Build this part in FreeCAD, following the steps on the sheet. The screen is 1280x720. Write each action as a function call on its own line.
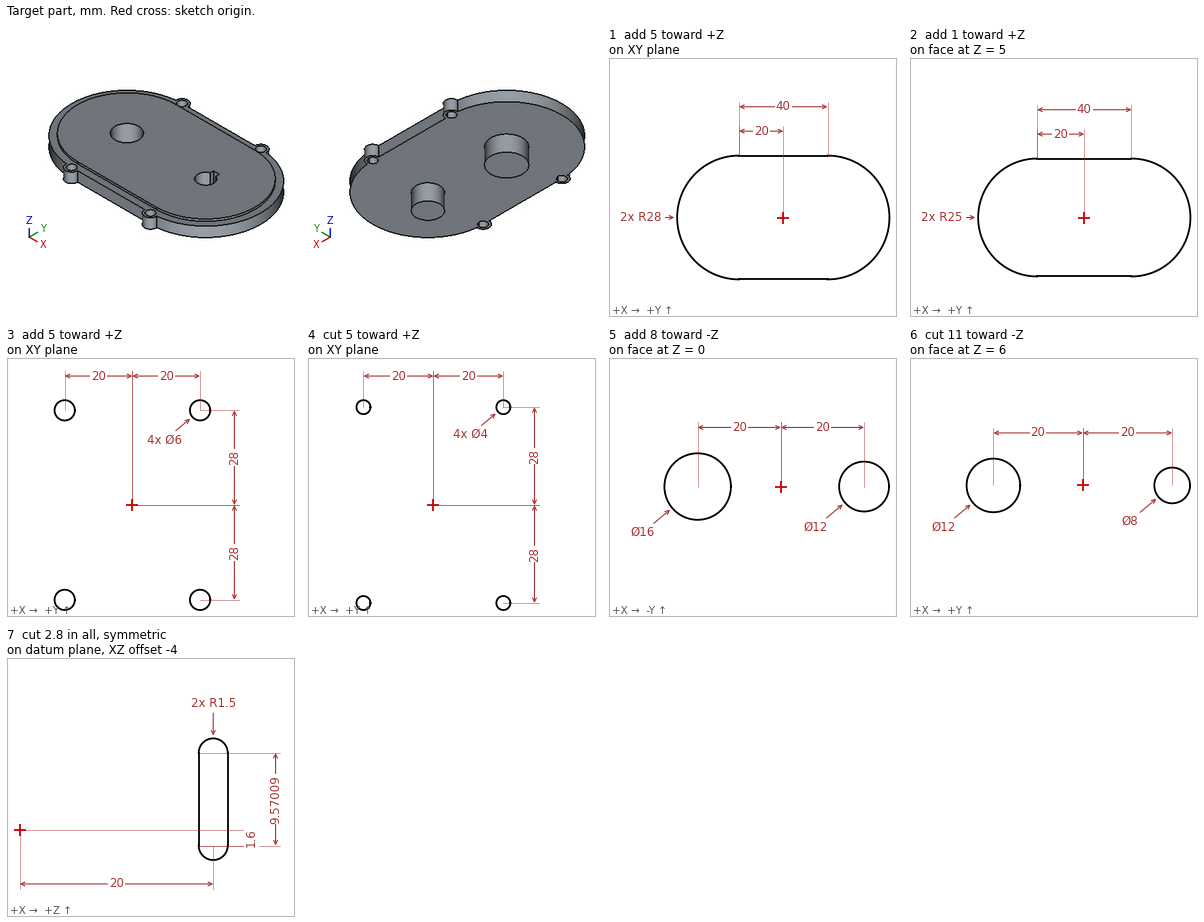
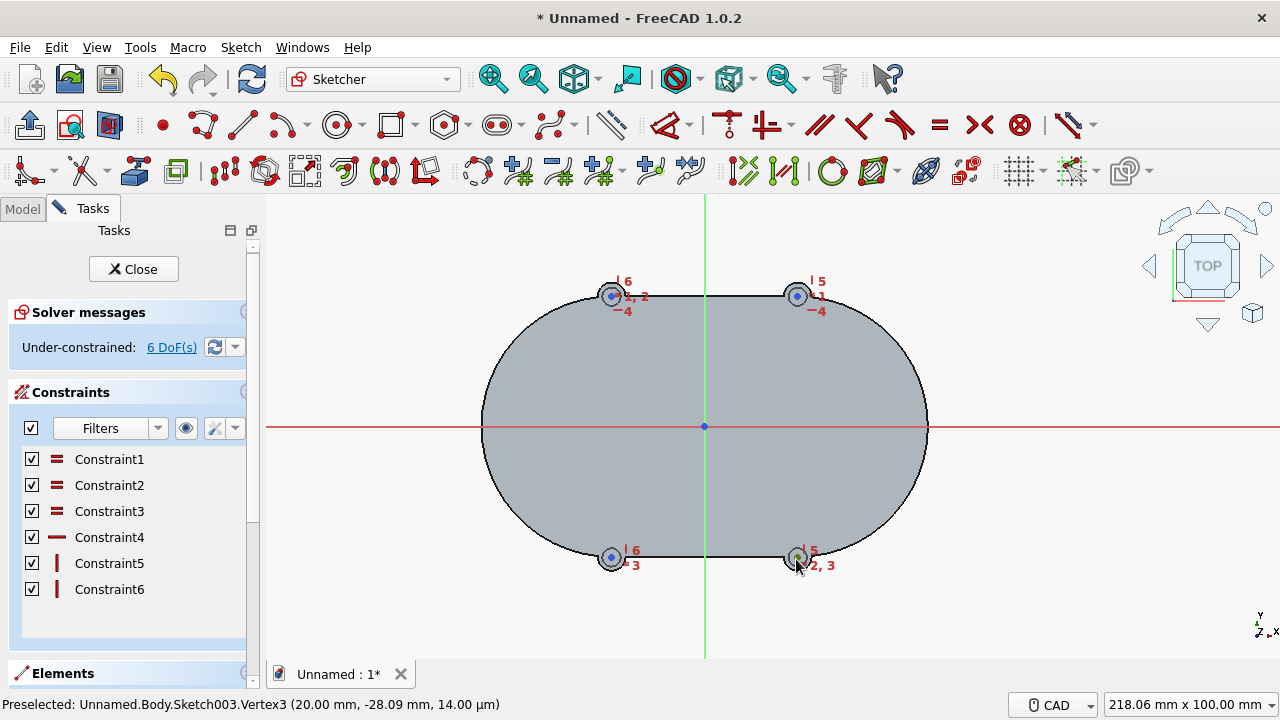
click(612, 557)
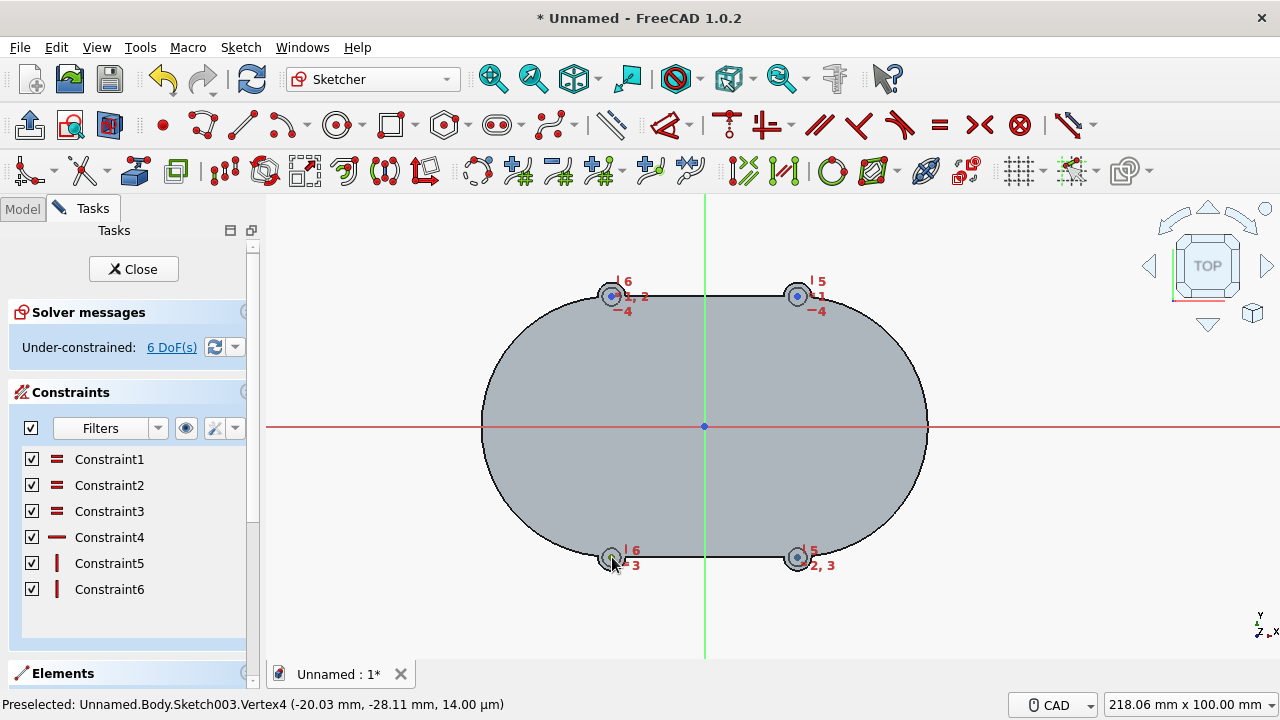
key(h)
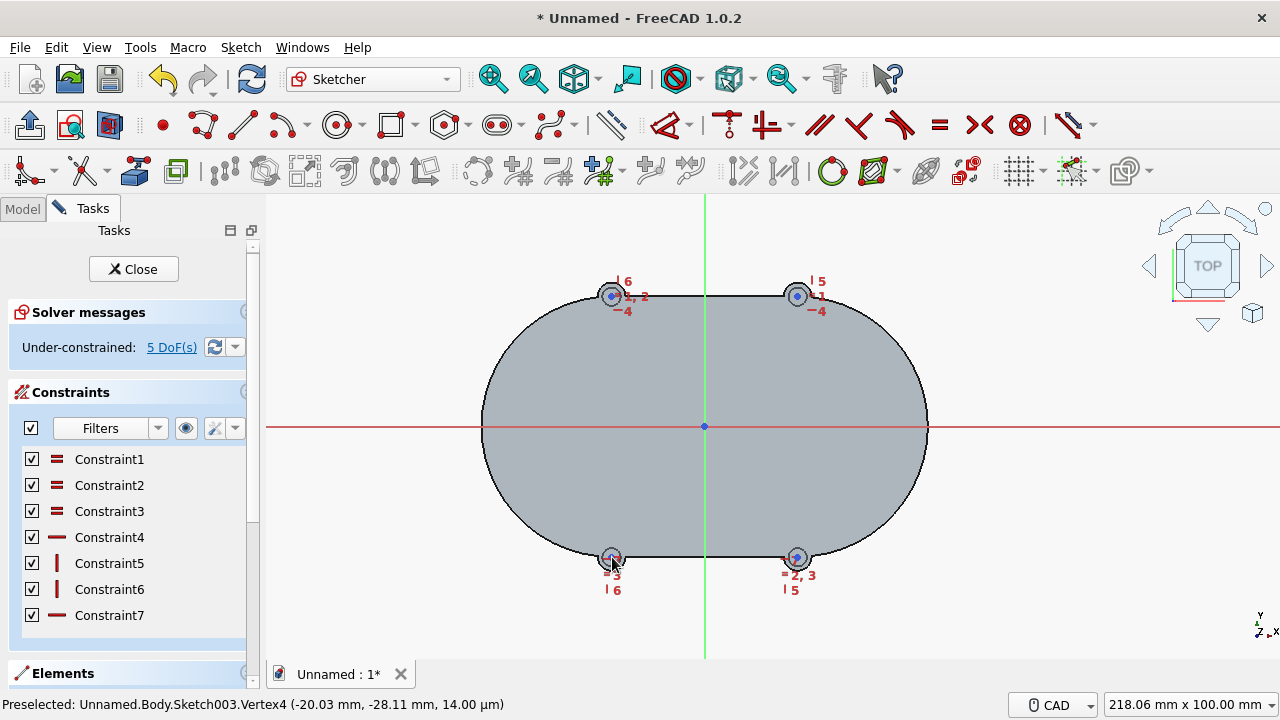
key(d)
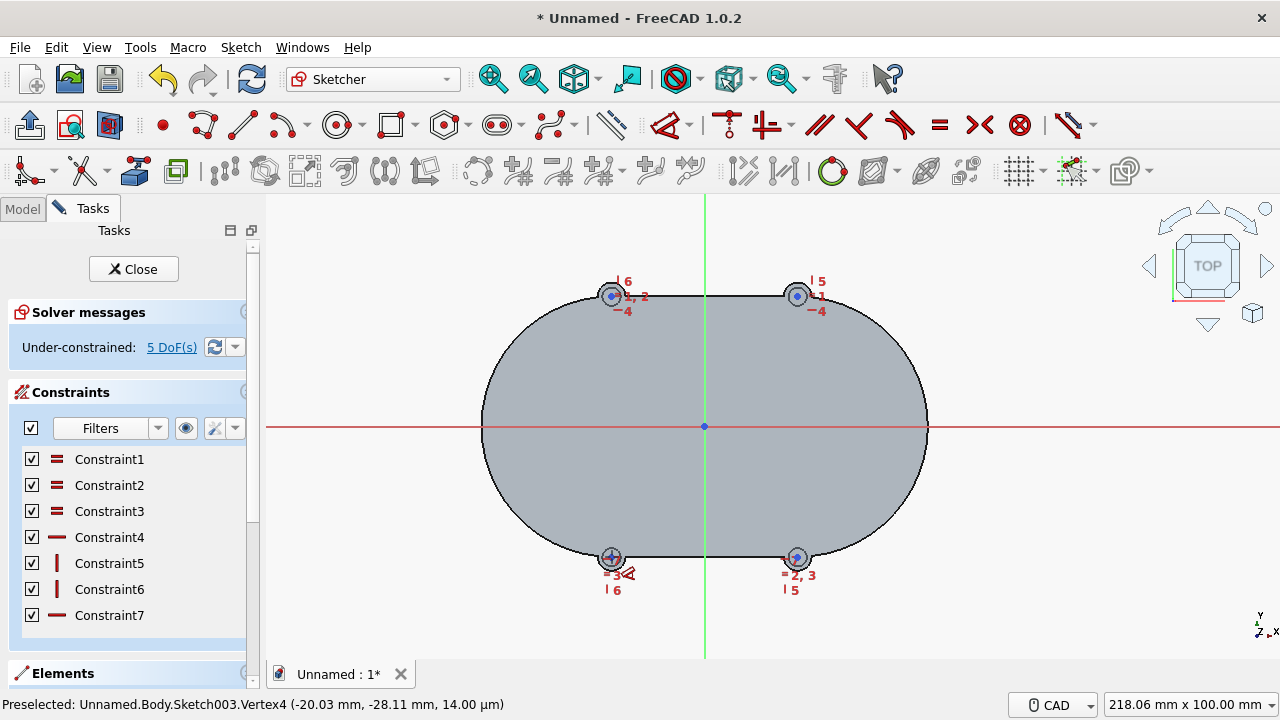
scroll(804, 290, up, 4)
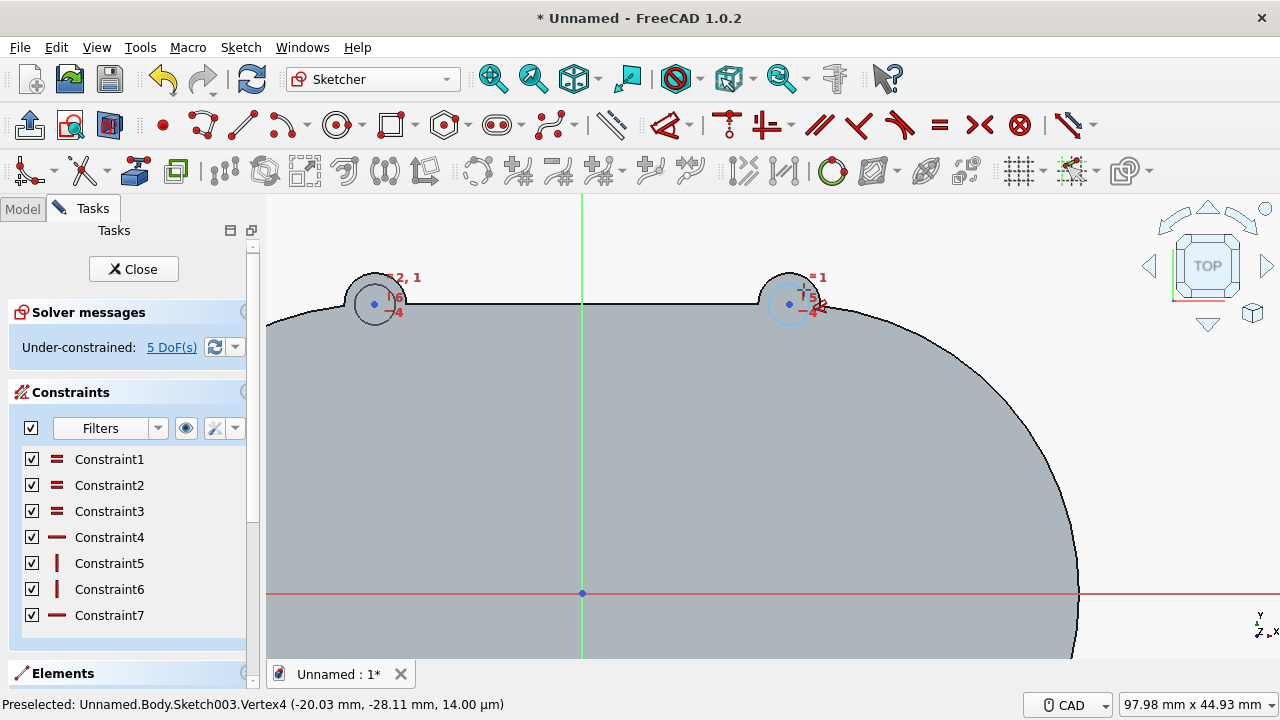
click(804, 290)
click(827, 267)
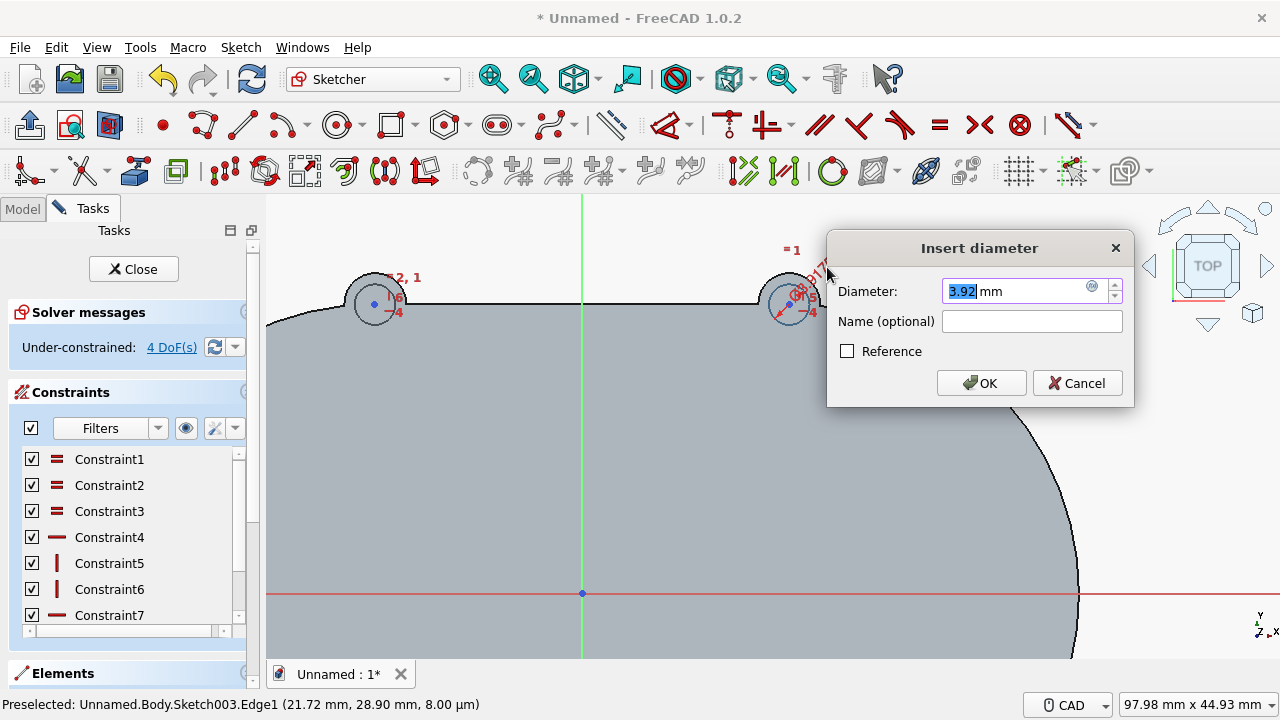
text(4)
key(Return)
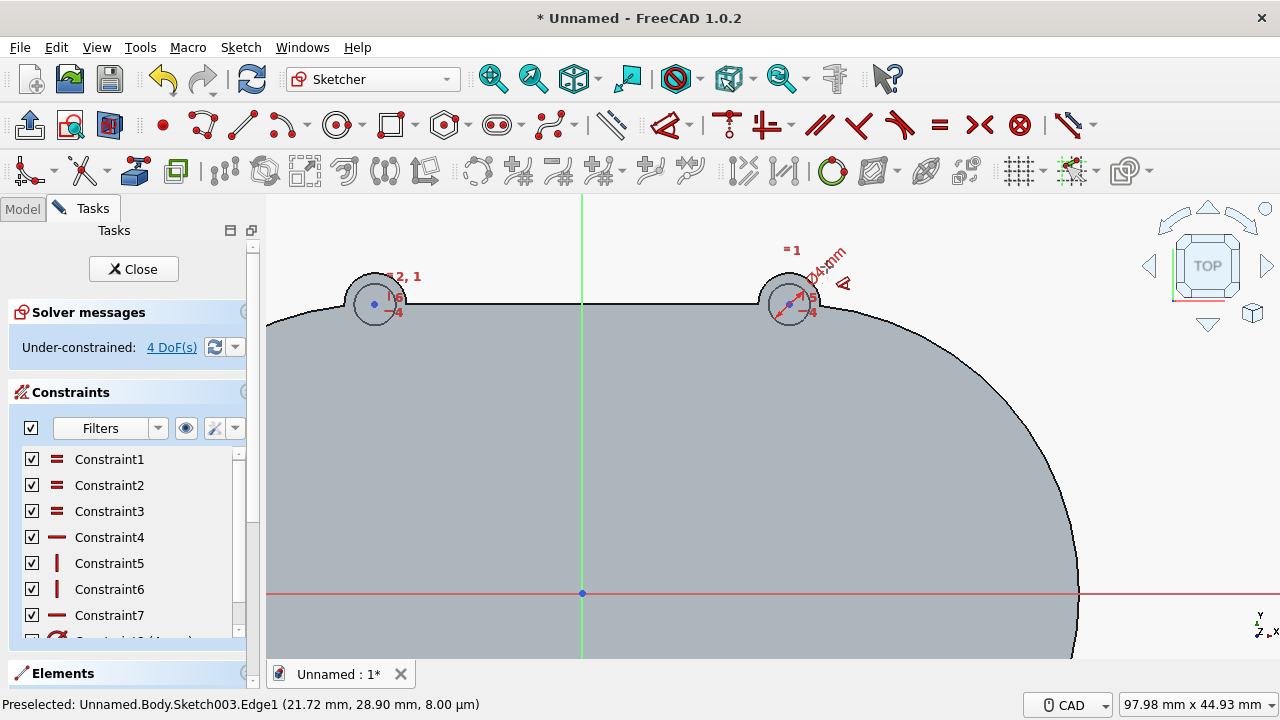
click(789, 305)
click(686, 271)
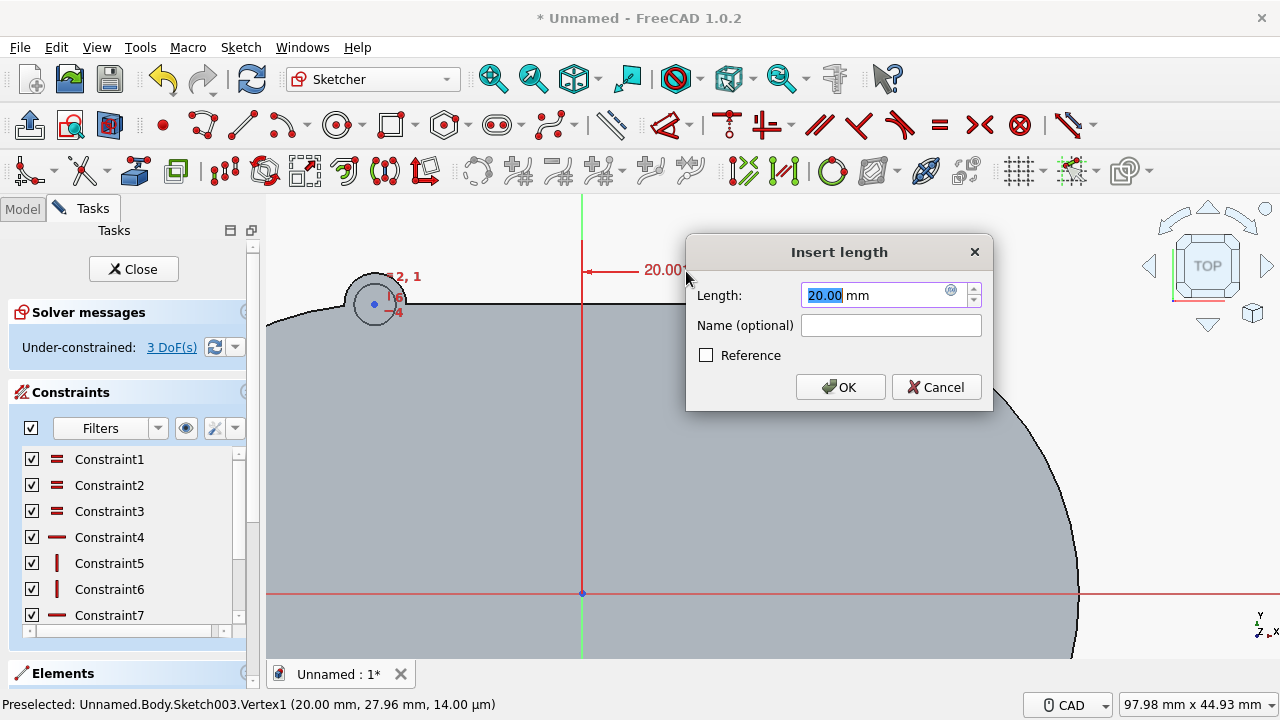
text(20)
key(Return)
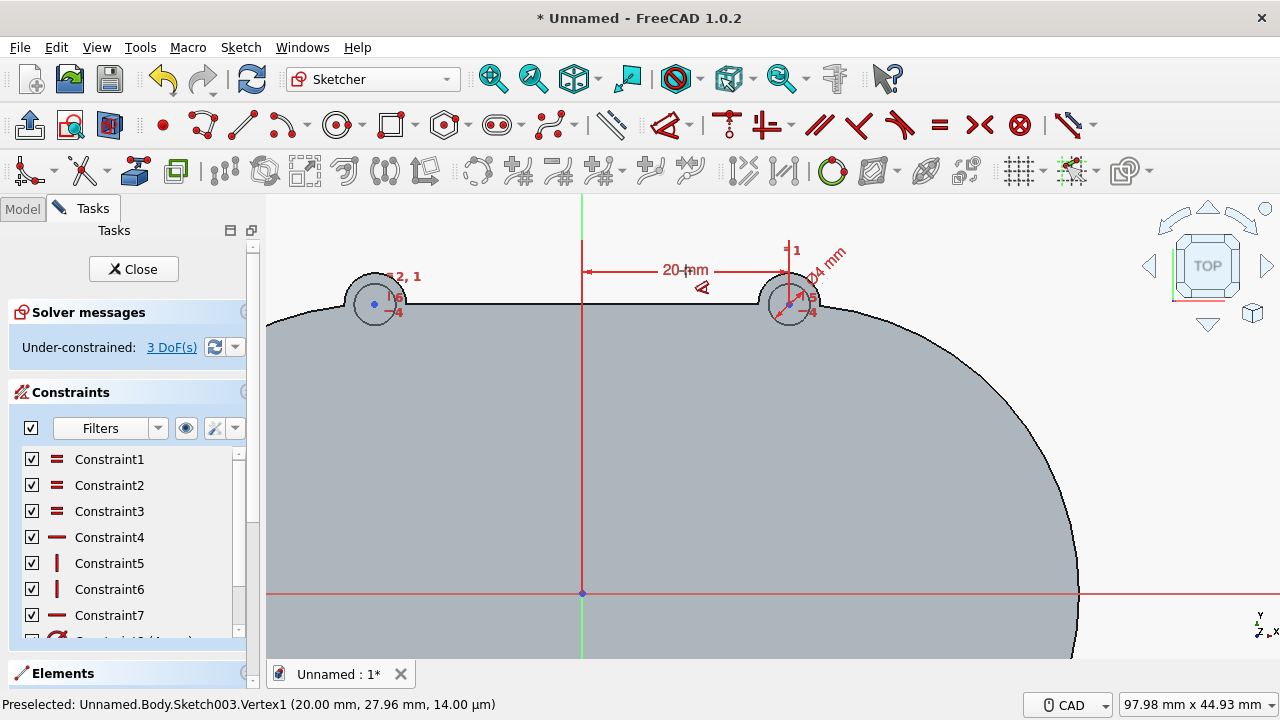
click(789, 305)
click(823, 449)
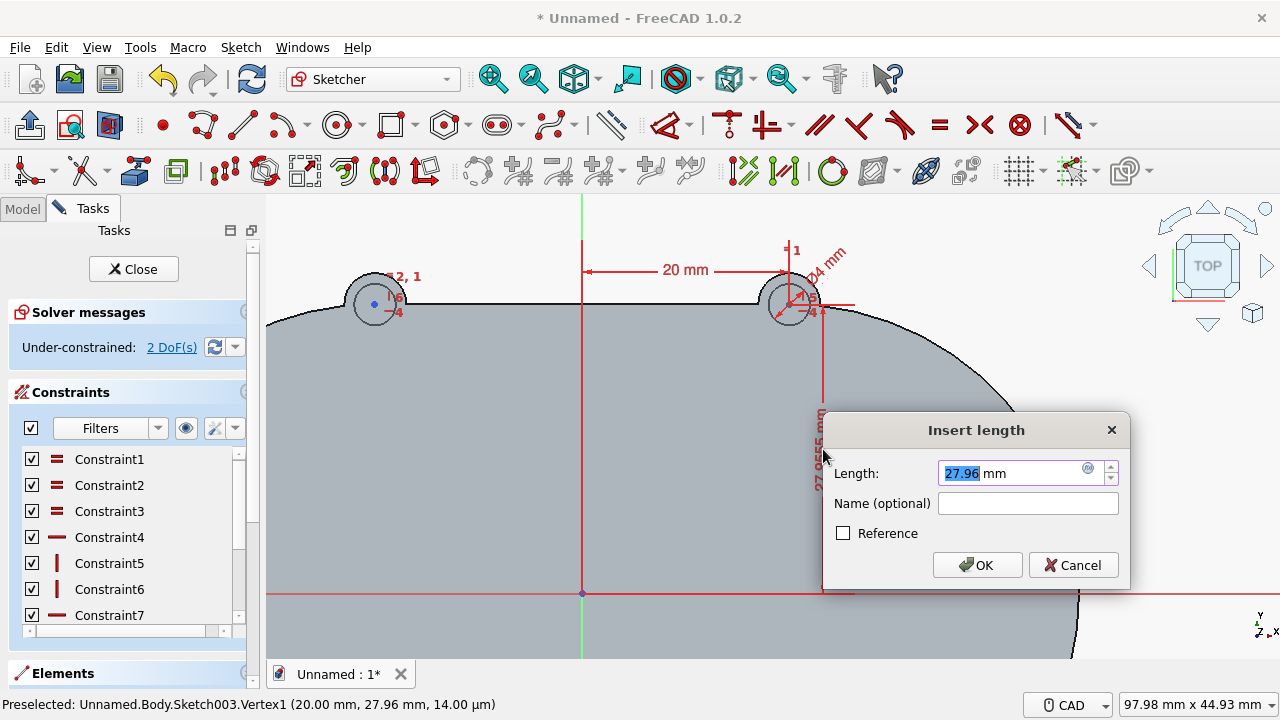
text(28)
key(Return)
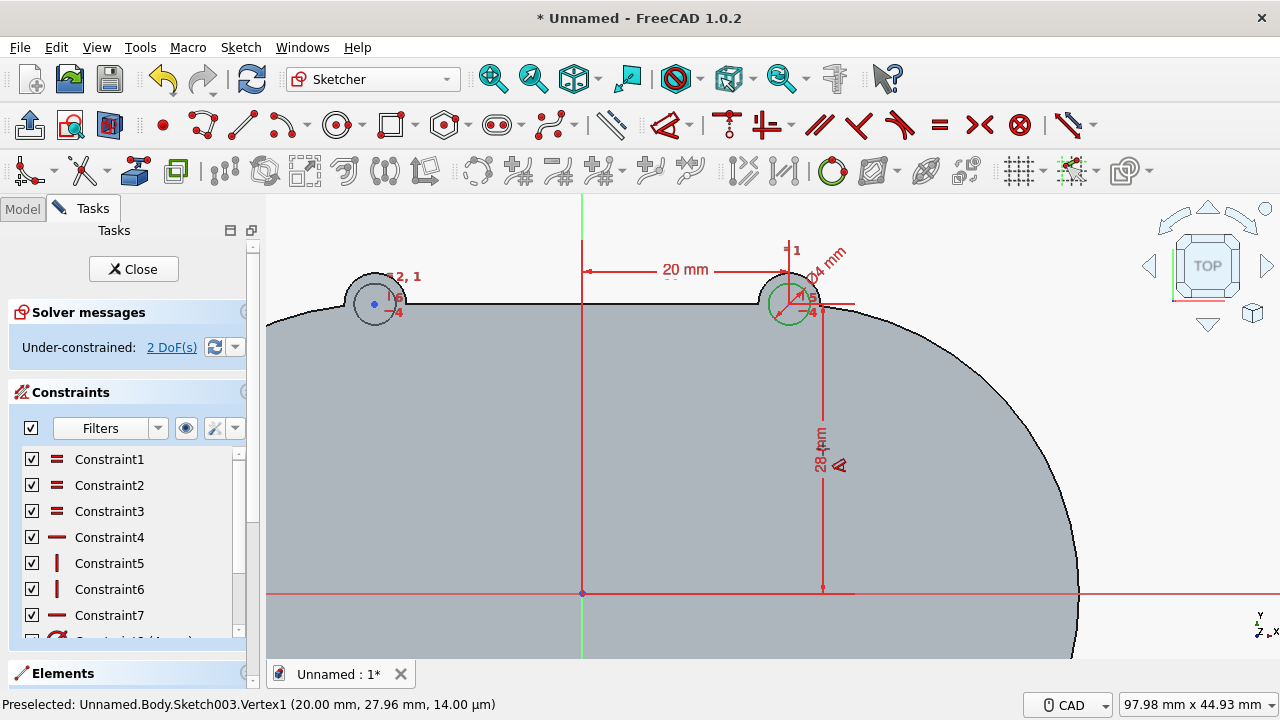
click(375, 304)
click(479, 270)